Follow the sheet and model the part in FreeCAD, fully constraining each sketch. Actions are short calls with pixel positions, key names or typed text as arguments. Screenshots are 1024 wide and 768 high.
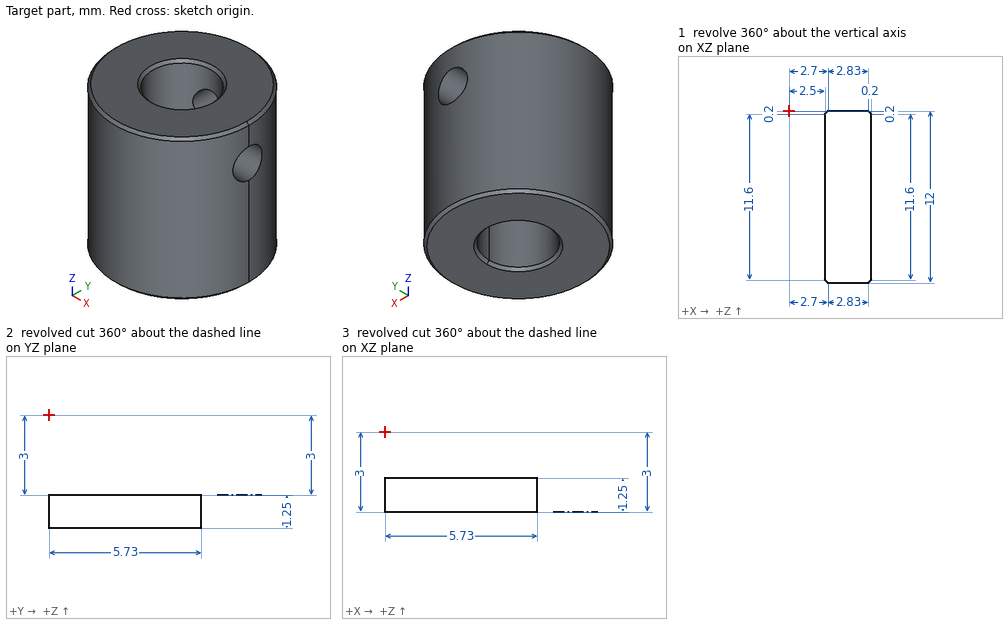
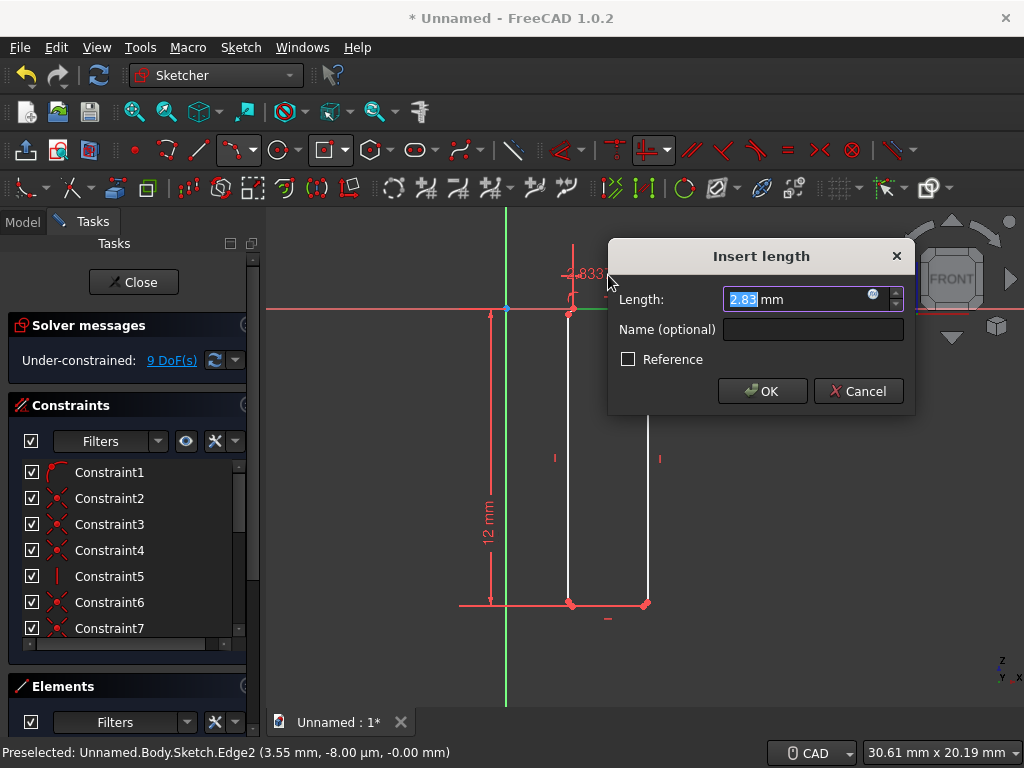
text(2.83)
key(Return)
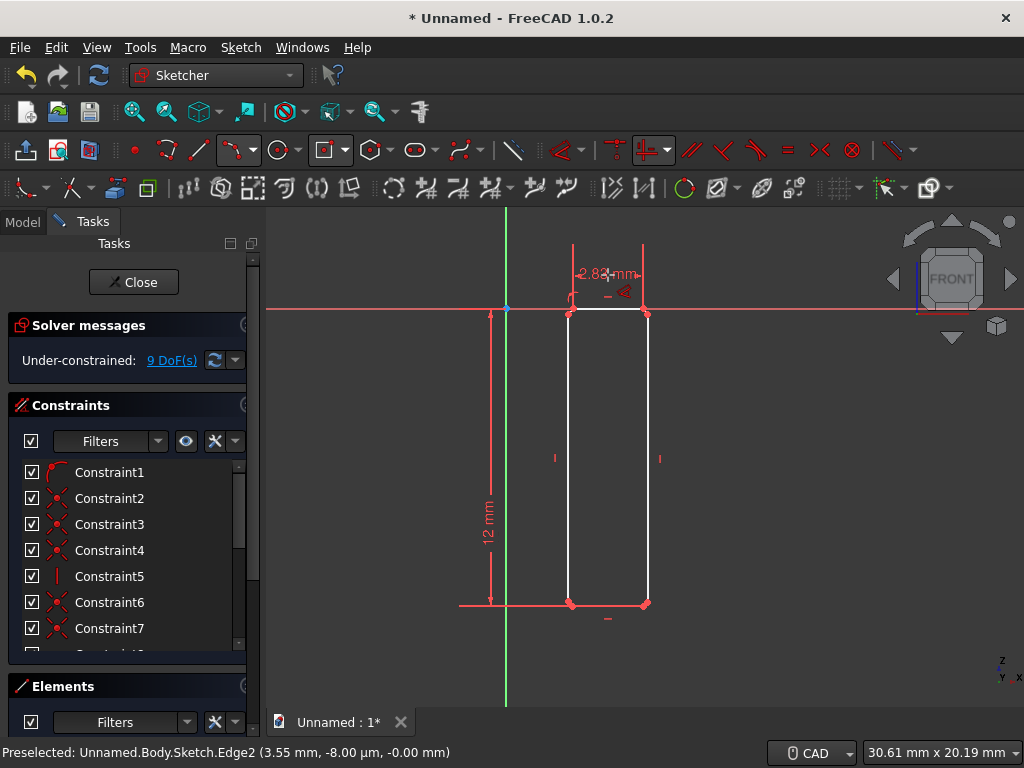
click(648, 401)
click(682, 458)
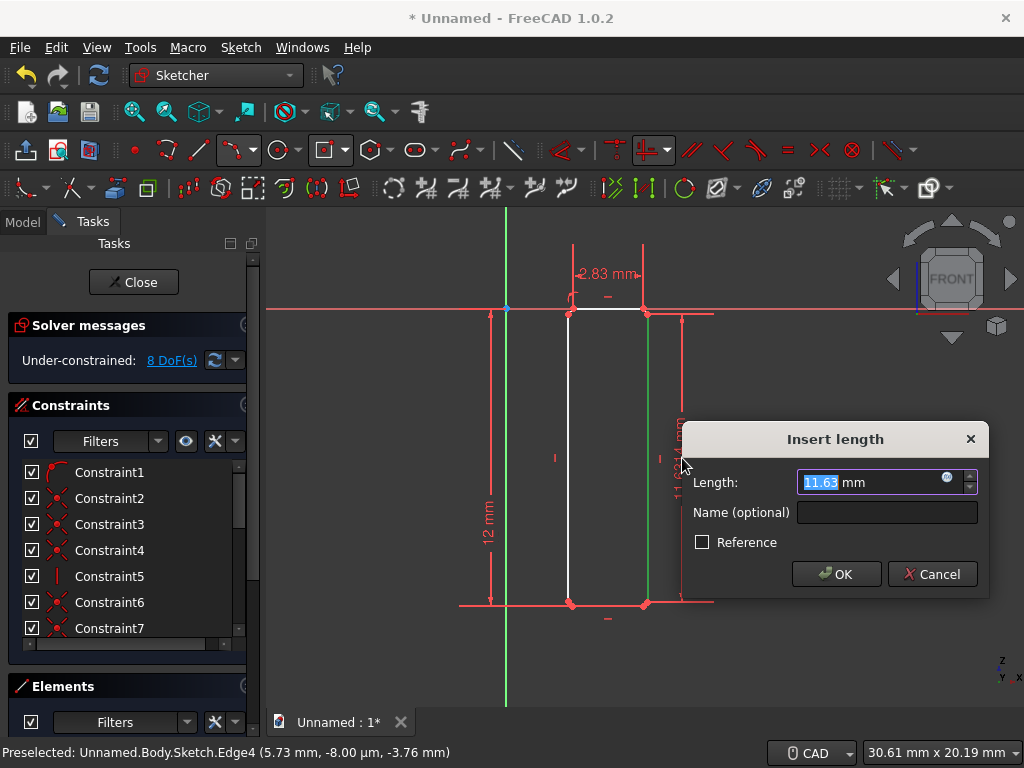
text(11.6)
key(Return)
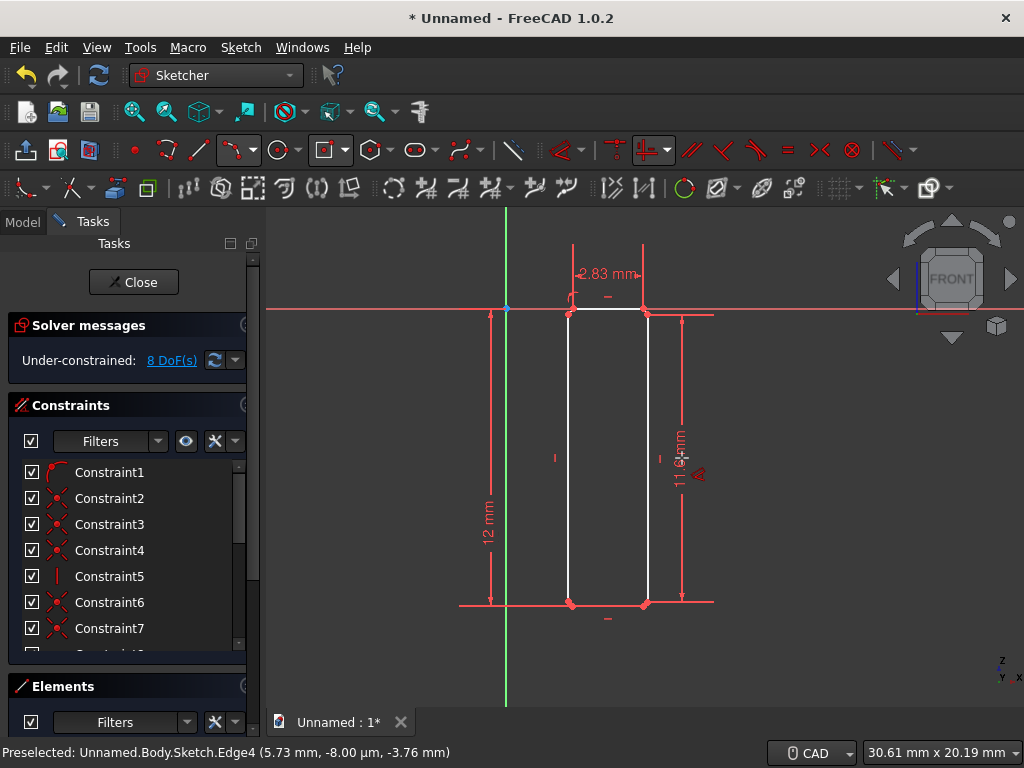
click(622, 606)
click(608, 640)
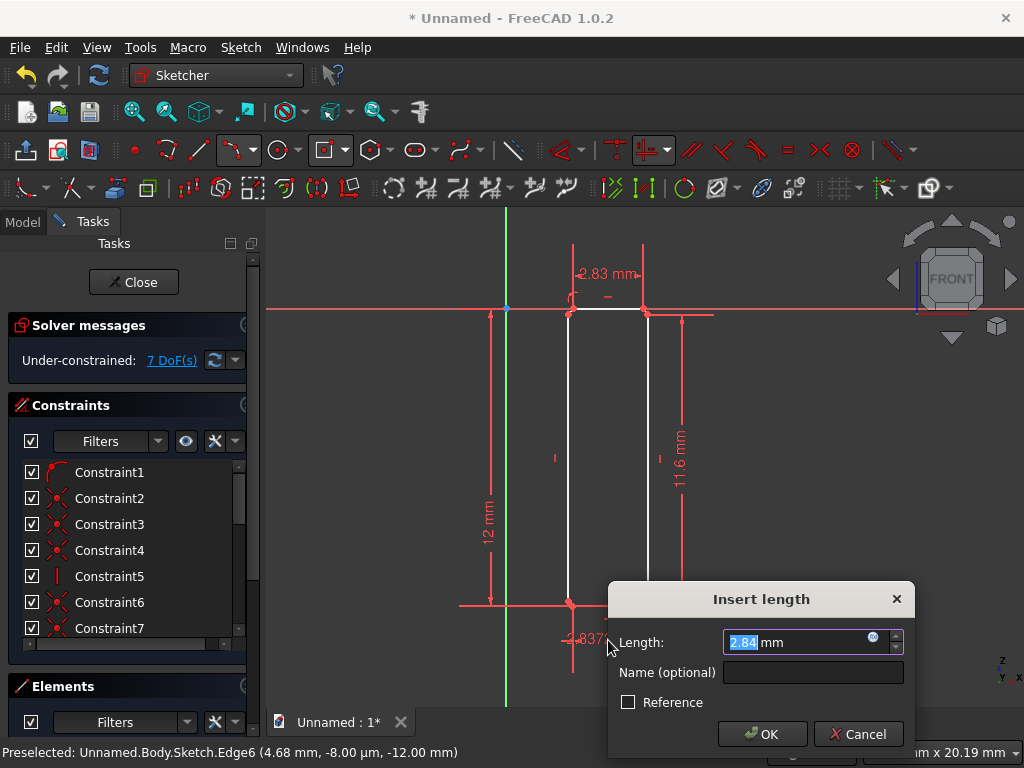
text(2.83)
key(Return)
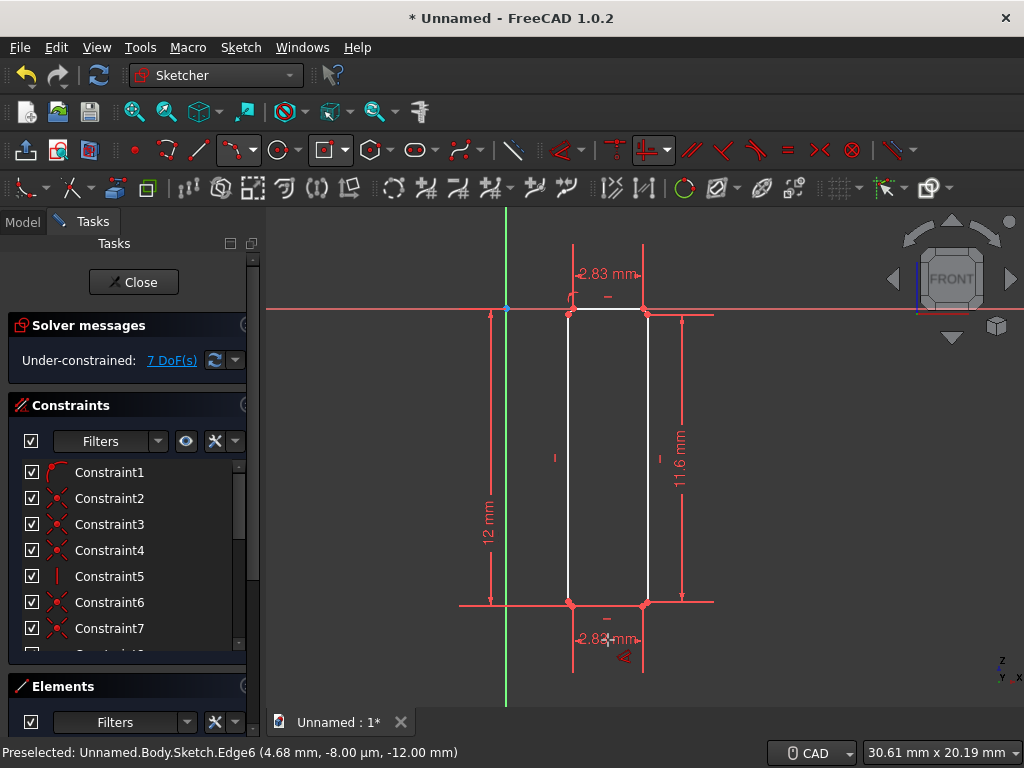
click(568, 515)
click(534, 458)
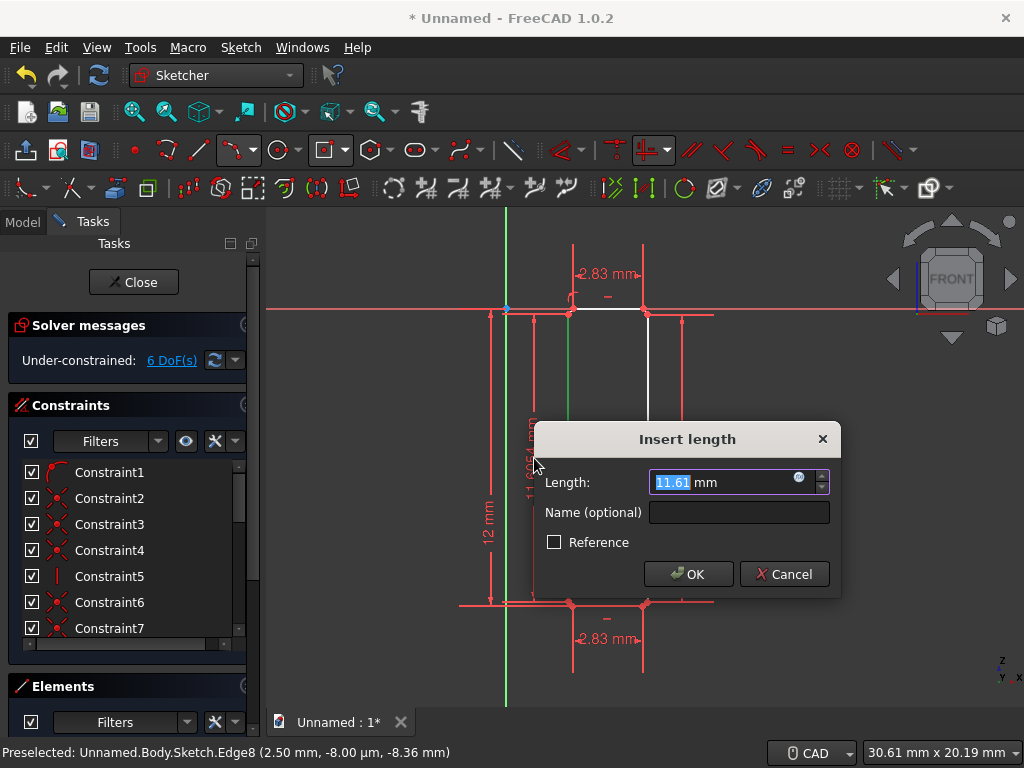
text(11.6)
key(Return)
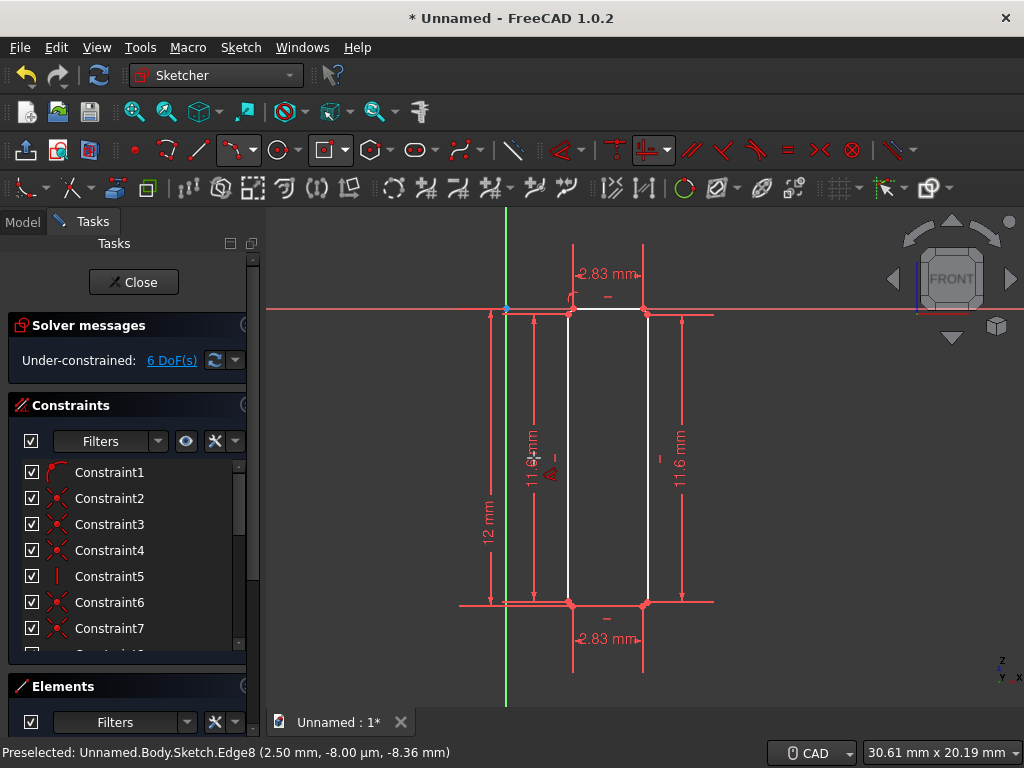
scroll(568, 314, up, 3)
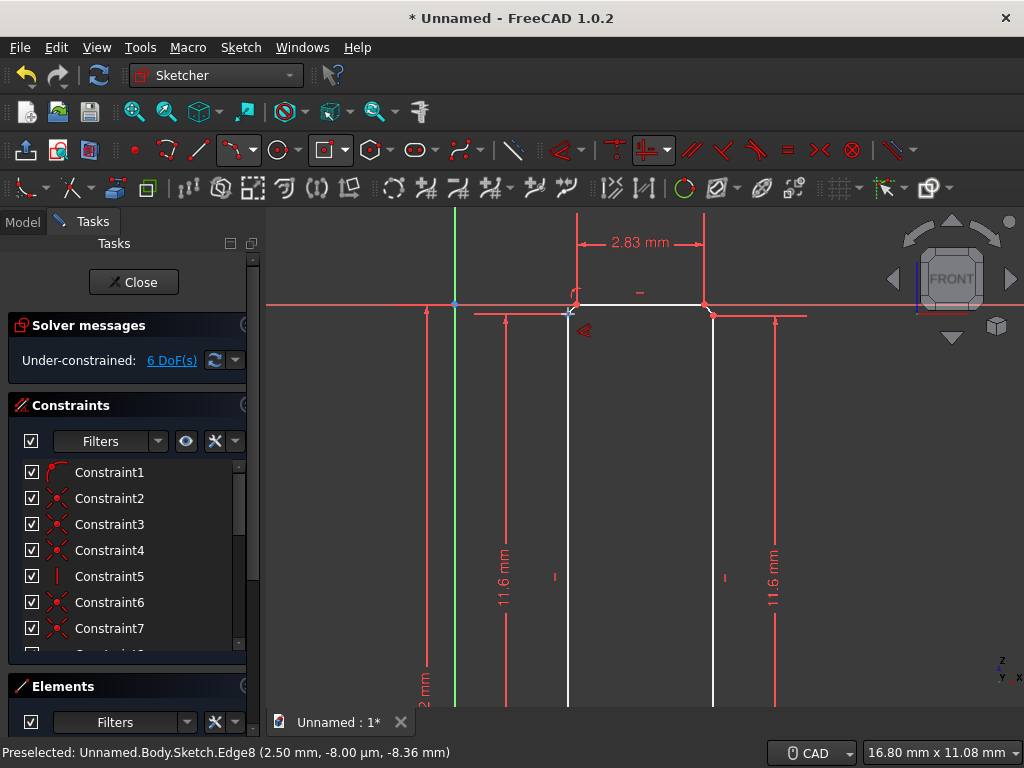
click(568, 314)
click(511, 271)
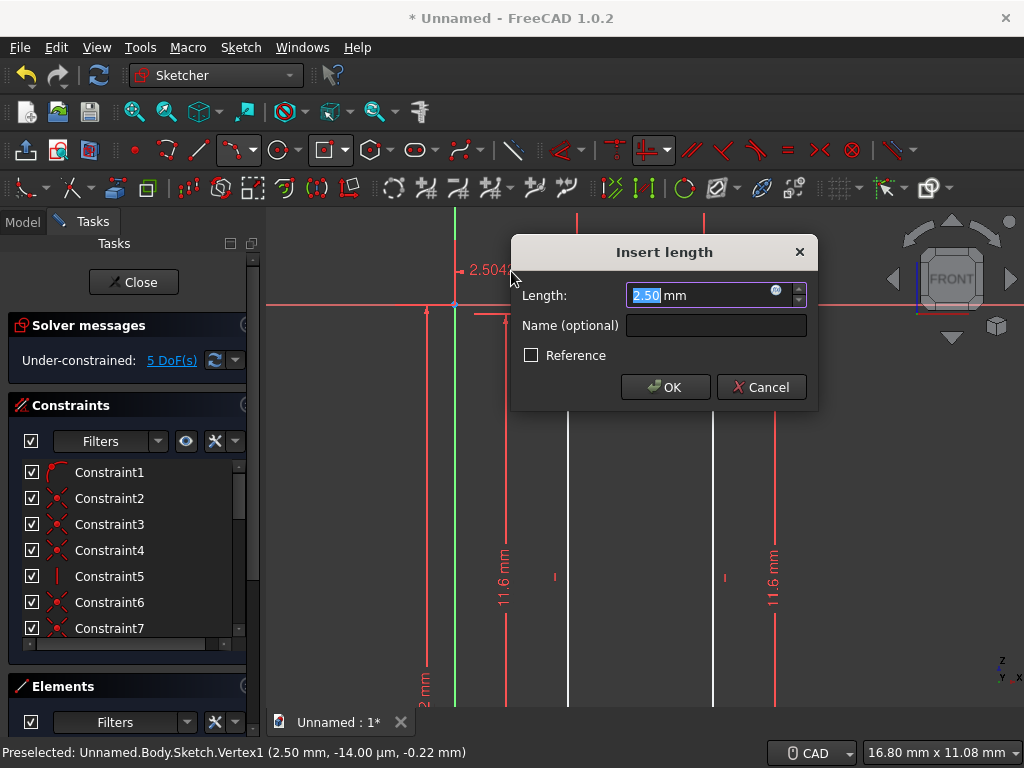
text(2.5)
key(Return)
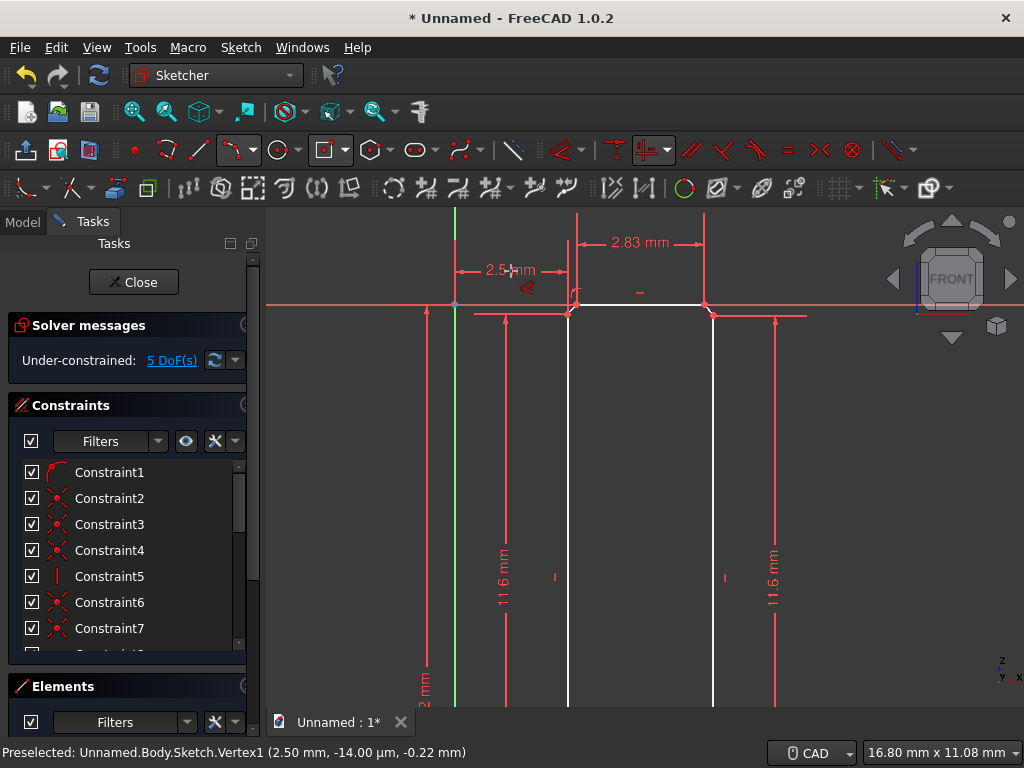
scroll(568, 314, up, 8)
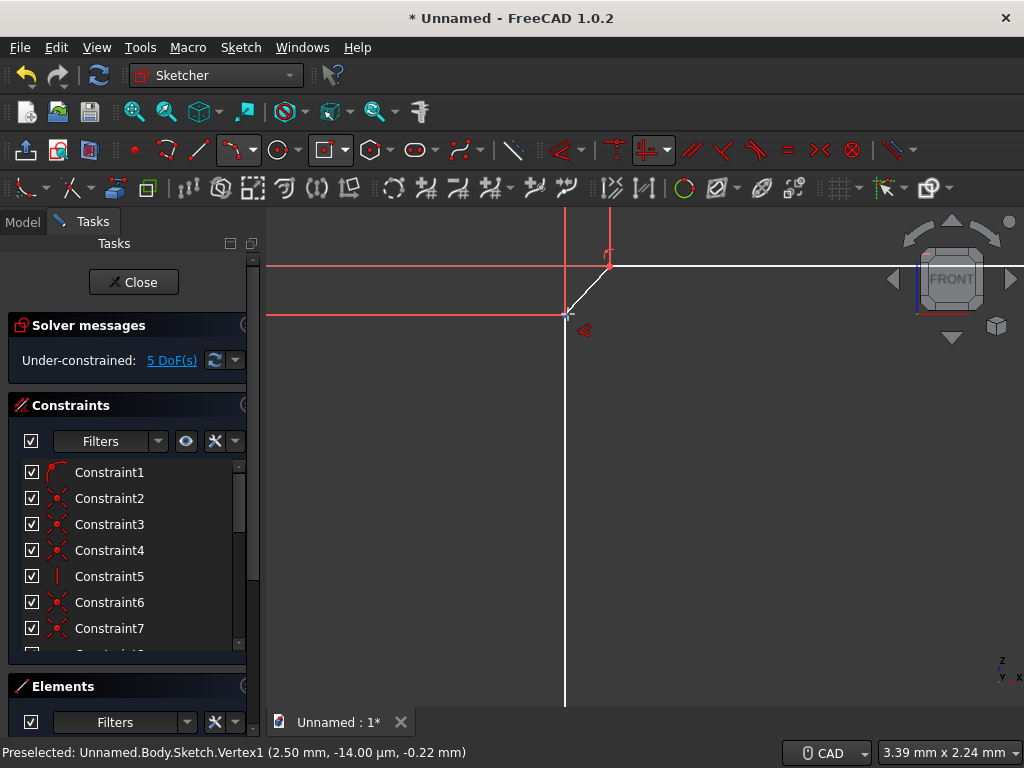
click(565, 315)
click(599, 302)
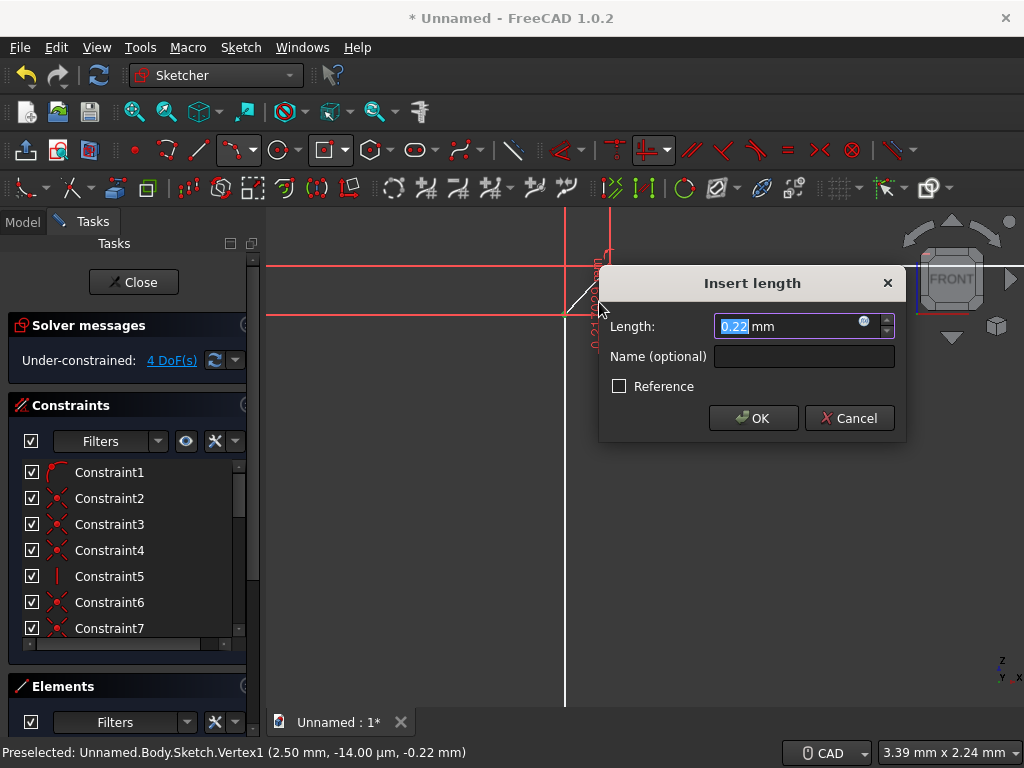
text(0.2)
key(Return)